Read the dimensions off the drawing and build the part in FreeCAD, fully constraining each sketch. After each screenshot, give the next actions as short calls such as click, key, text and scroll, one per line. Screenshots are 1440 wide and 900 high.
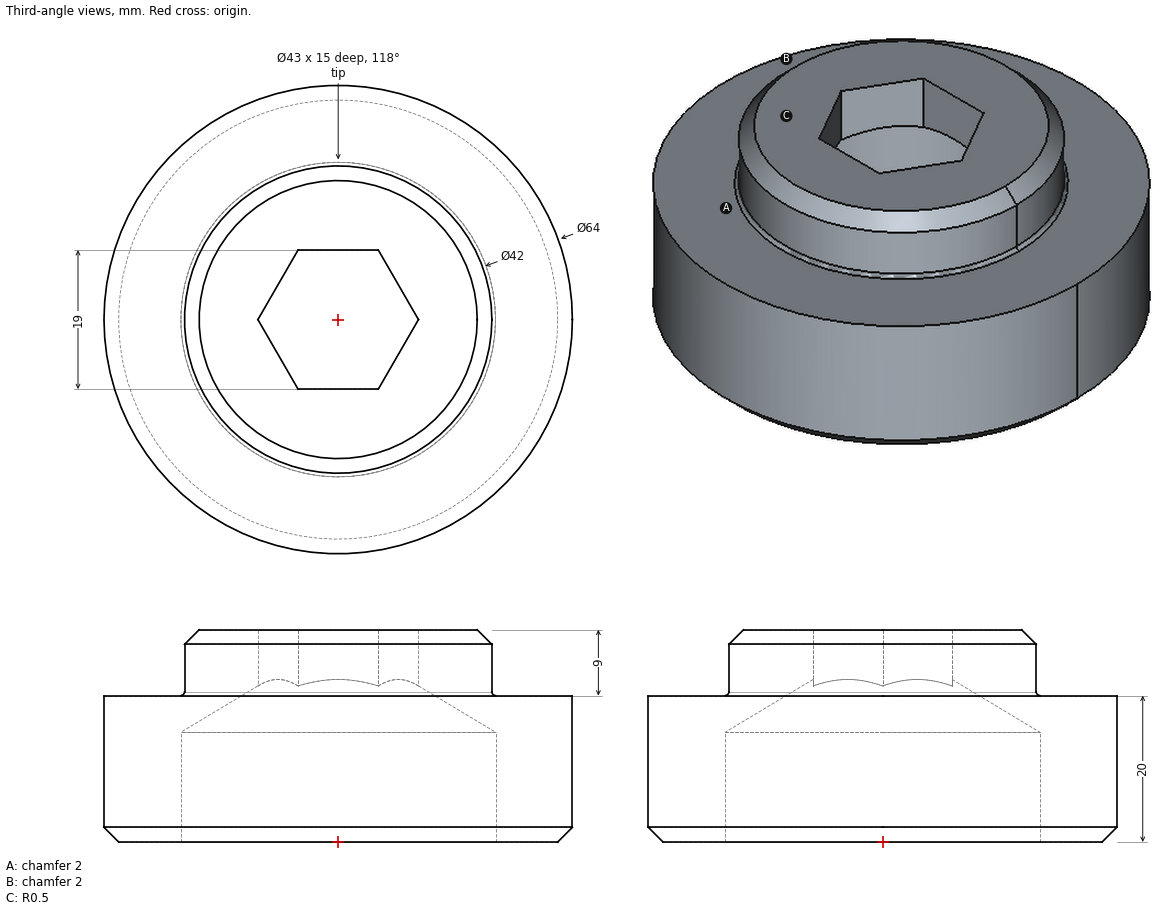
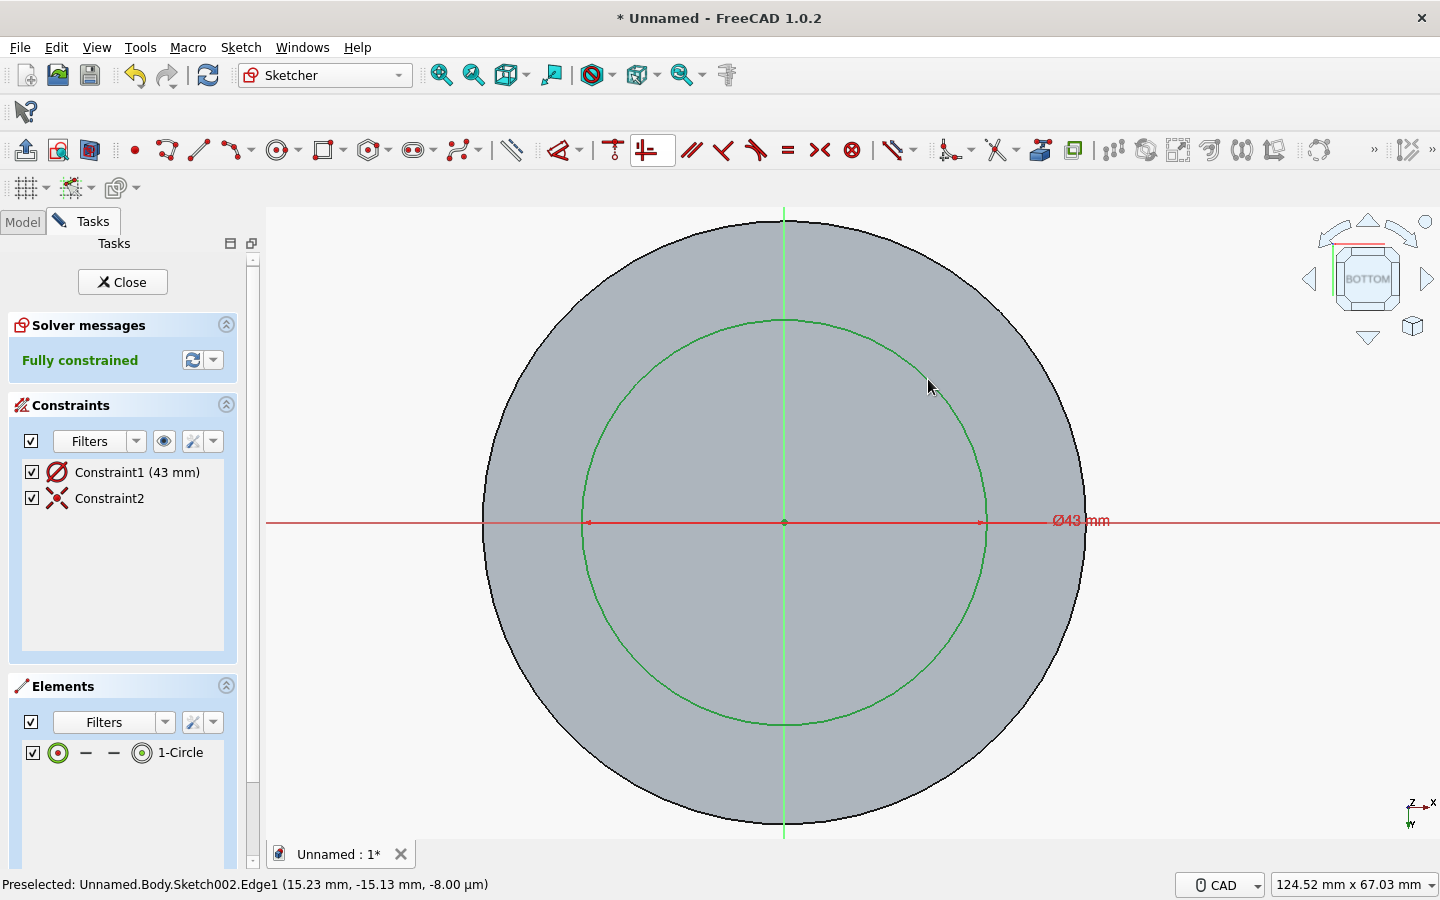
click(123, 282)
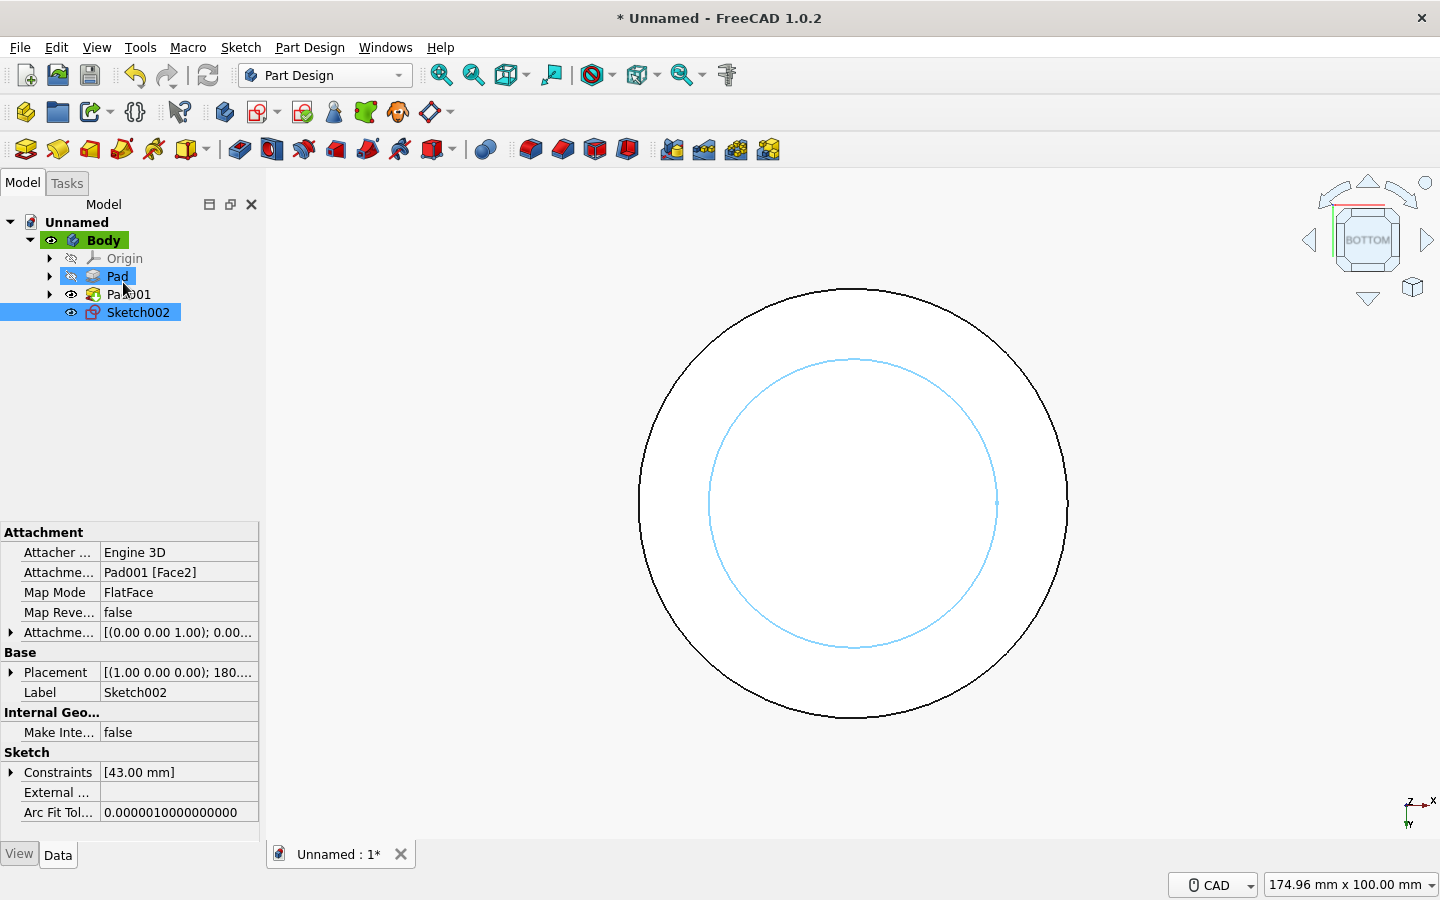
click(272, 150)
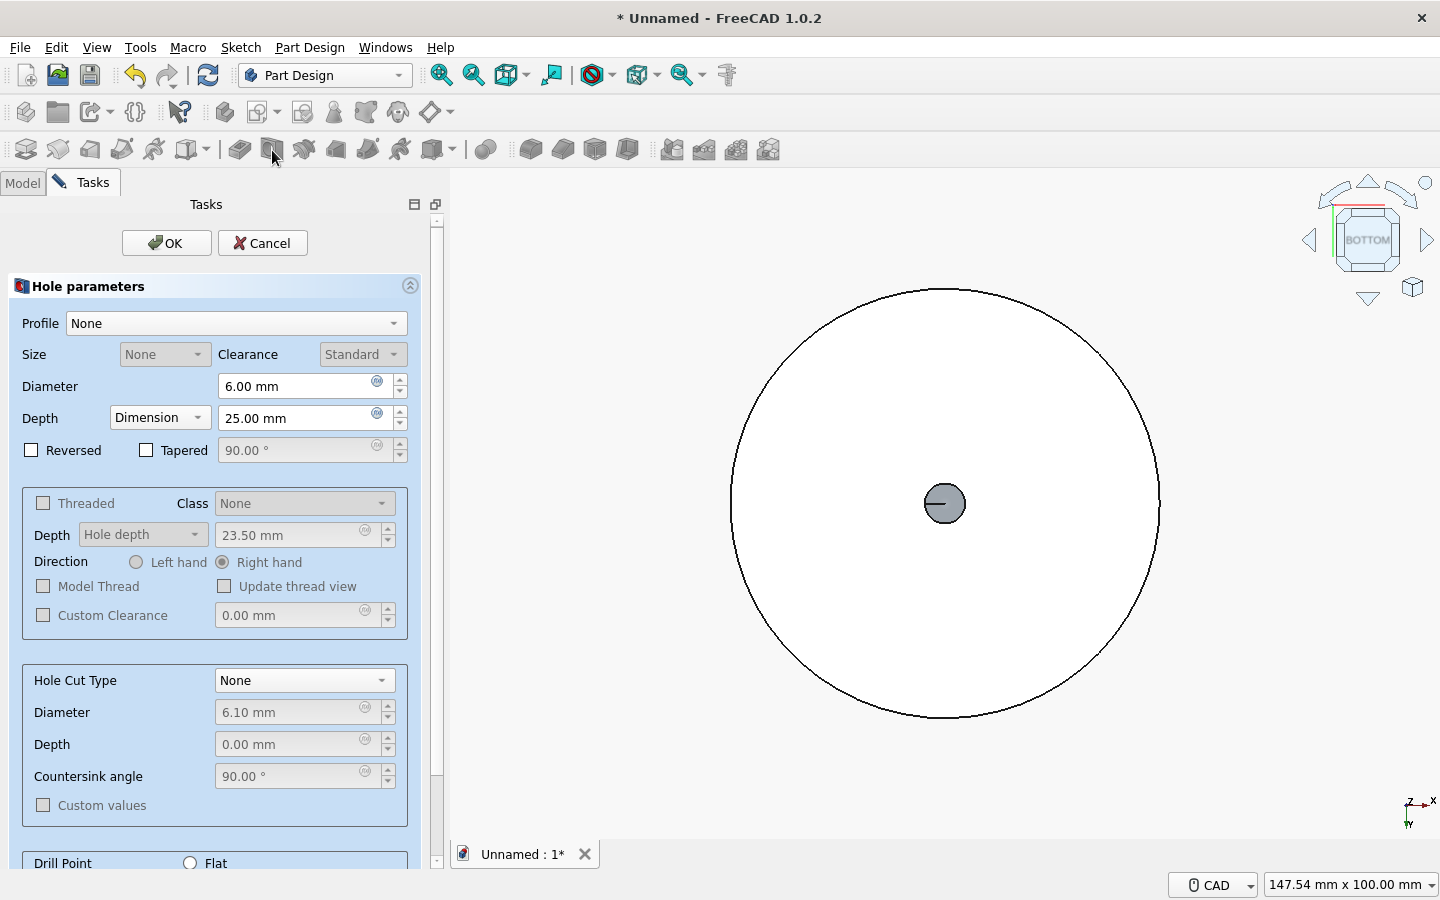
triple_click(305, 386)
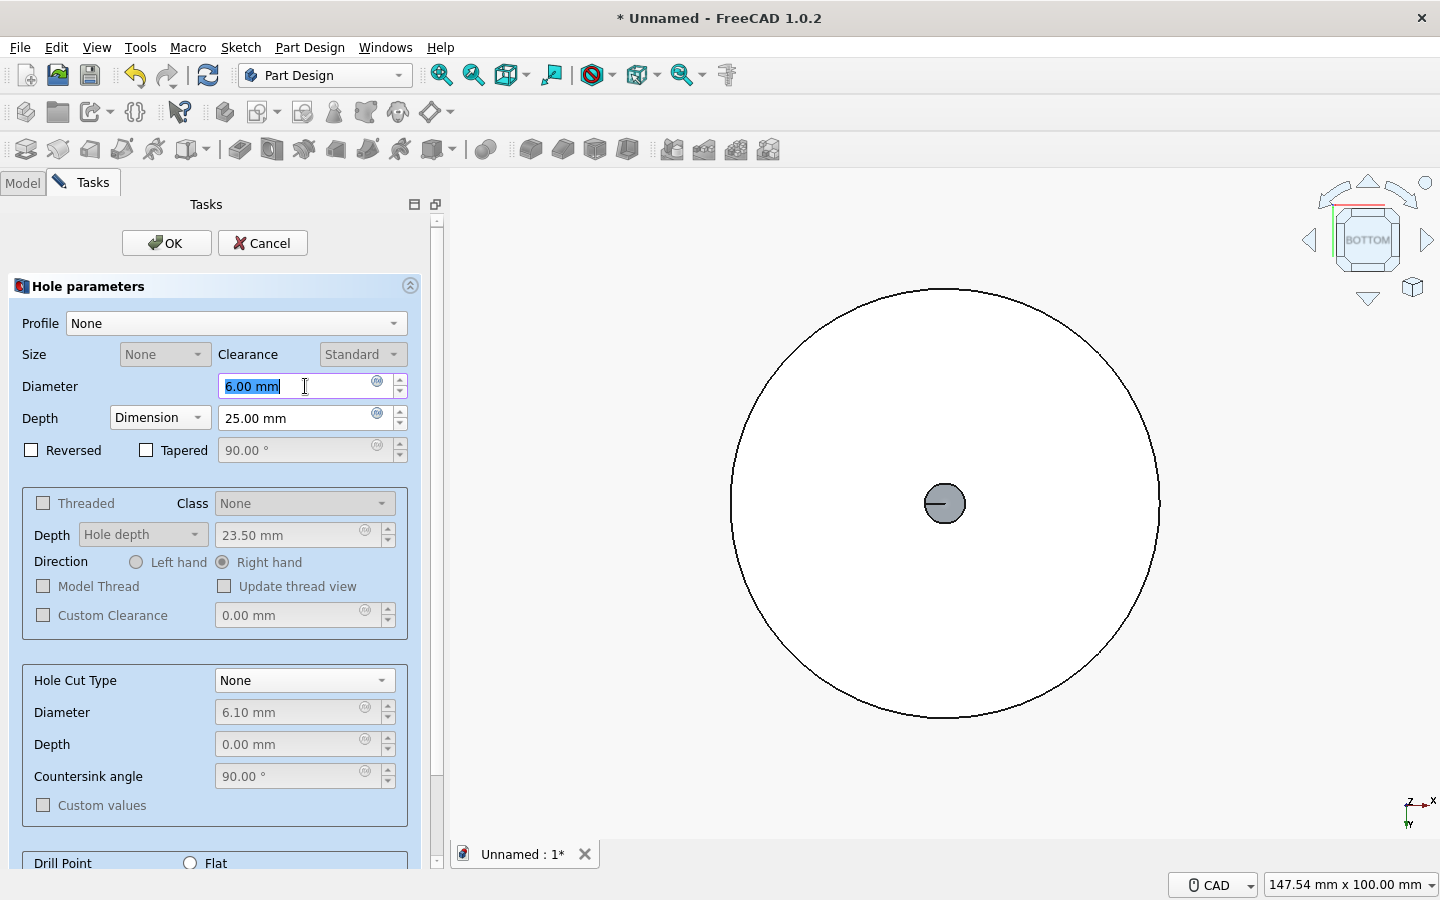
text(43)
key(Tab)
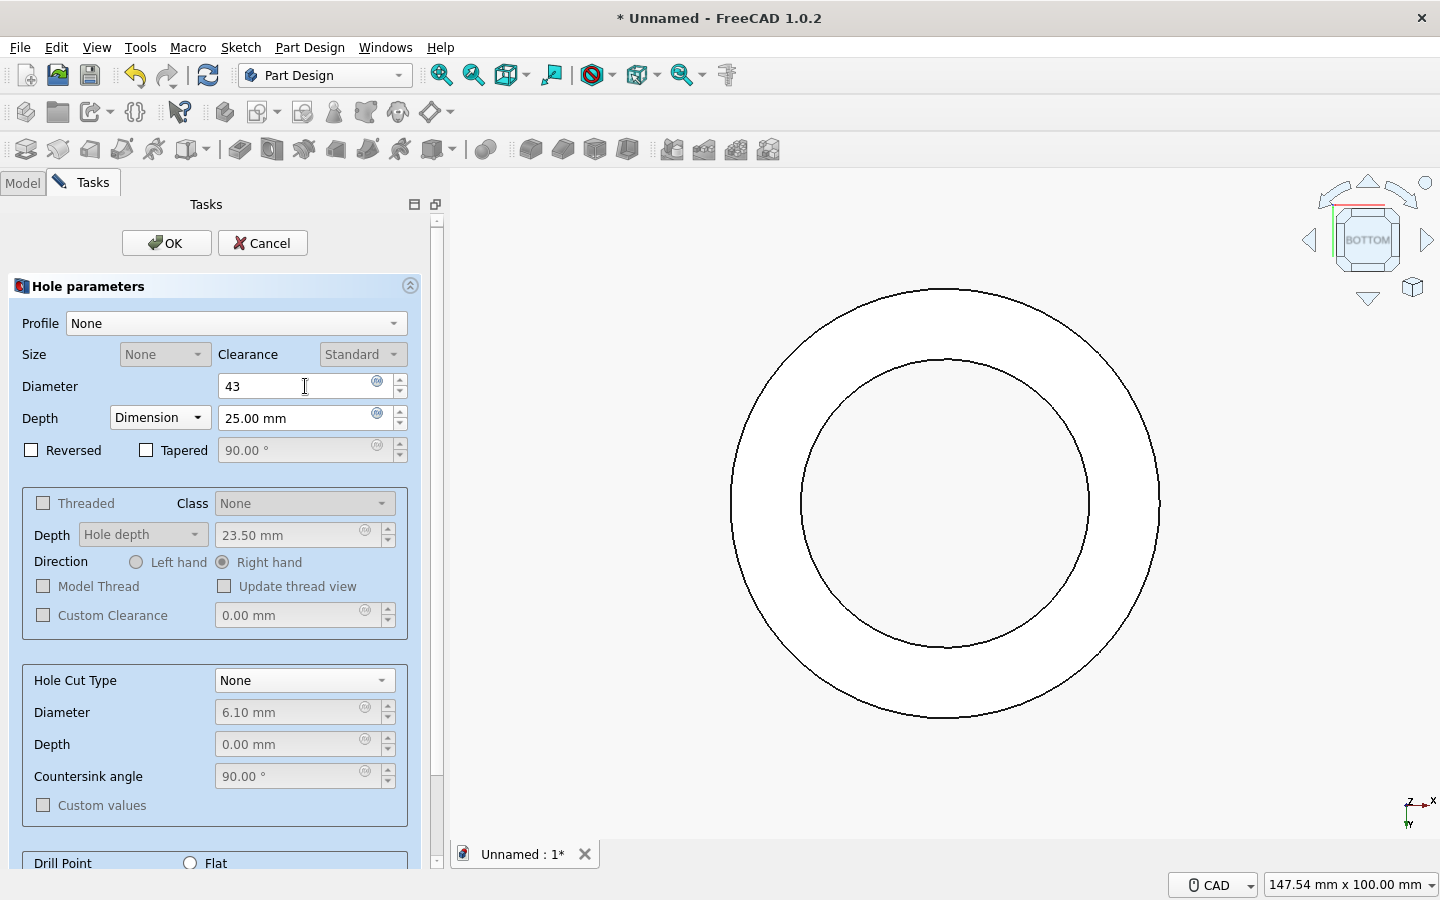
triple_click(305, 418)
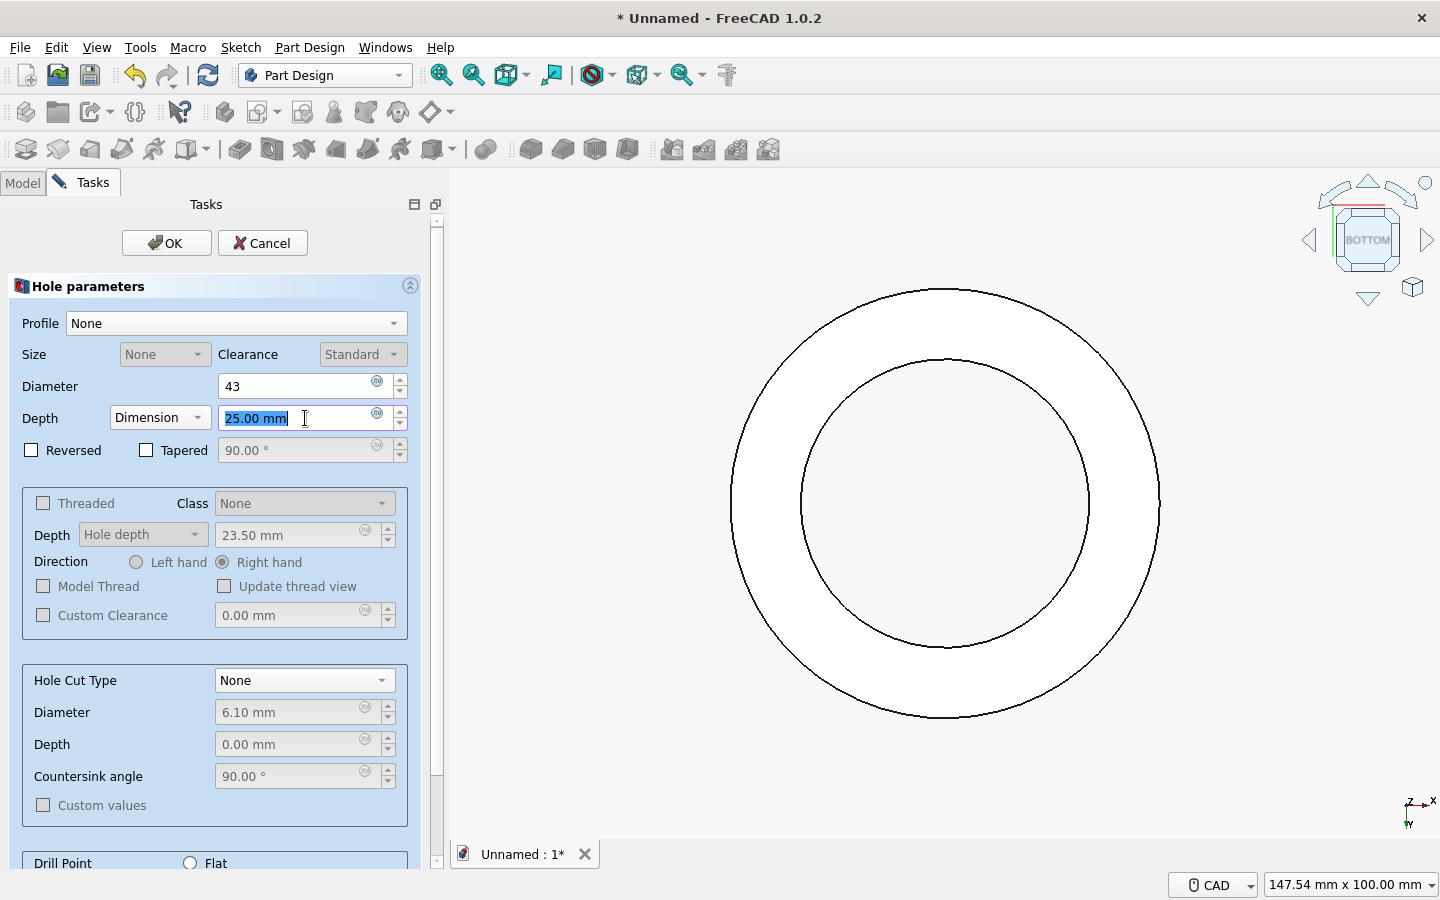
text(15)
key(Tab)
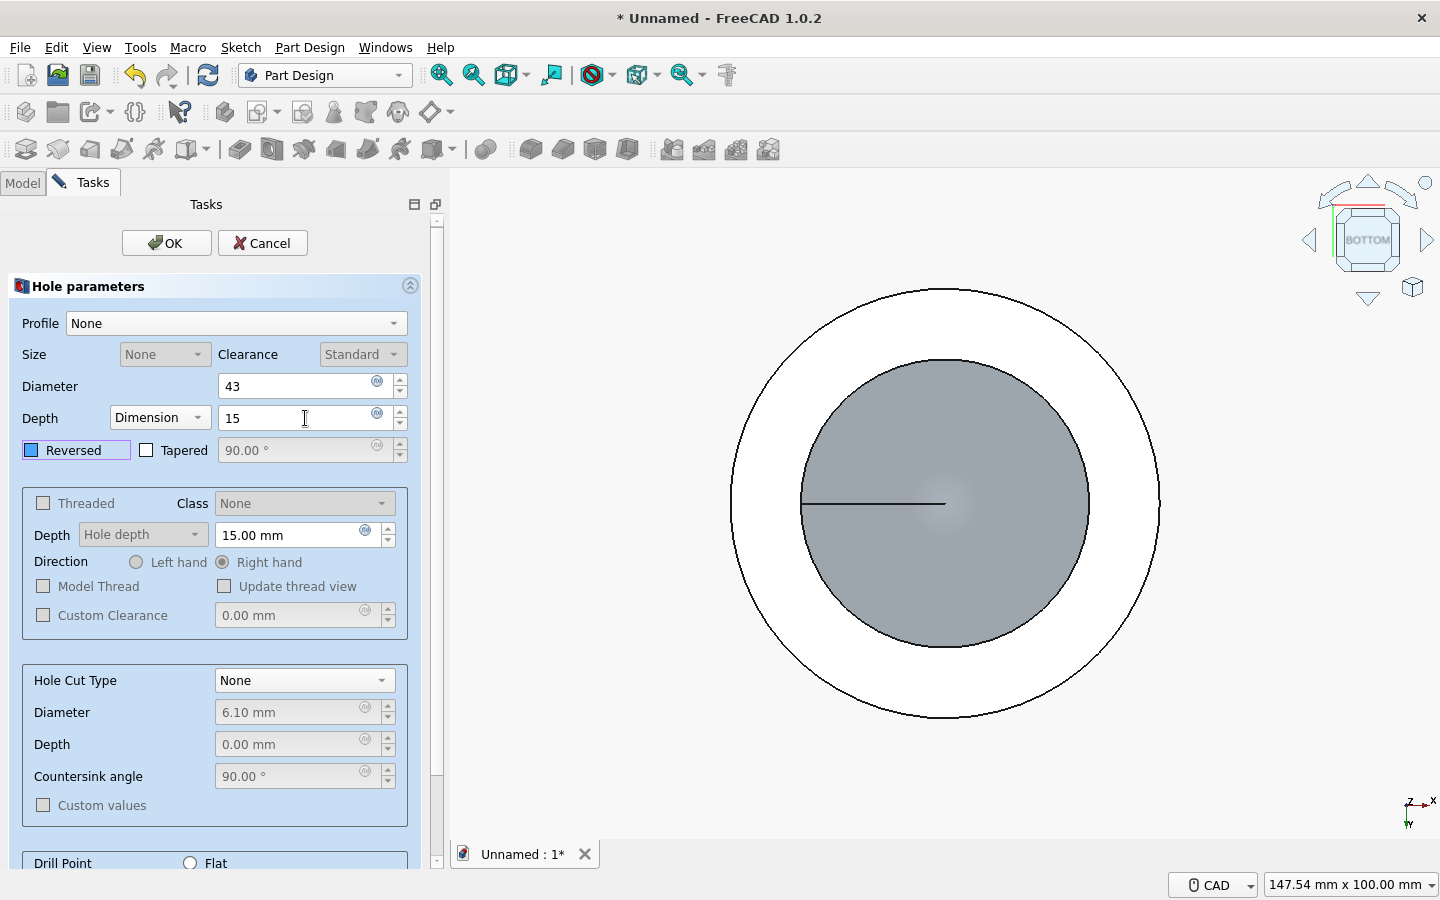
click(167, 243)